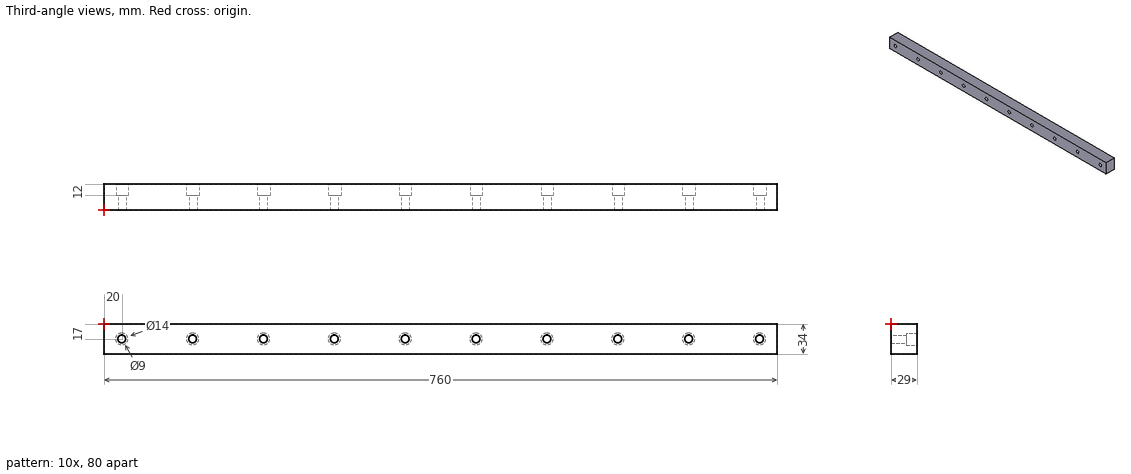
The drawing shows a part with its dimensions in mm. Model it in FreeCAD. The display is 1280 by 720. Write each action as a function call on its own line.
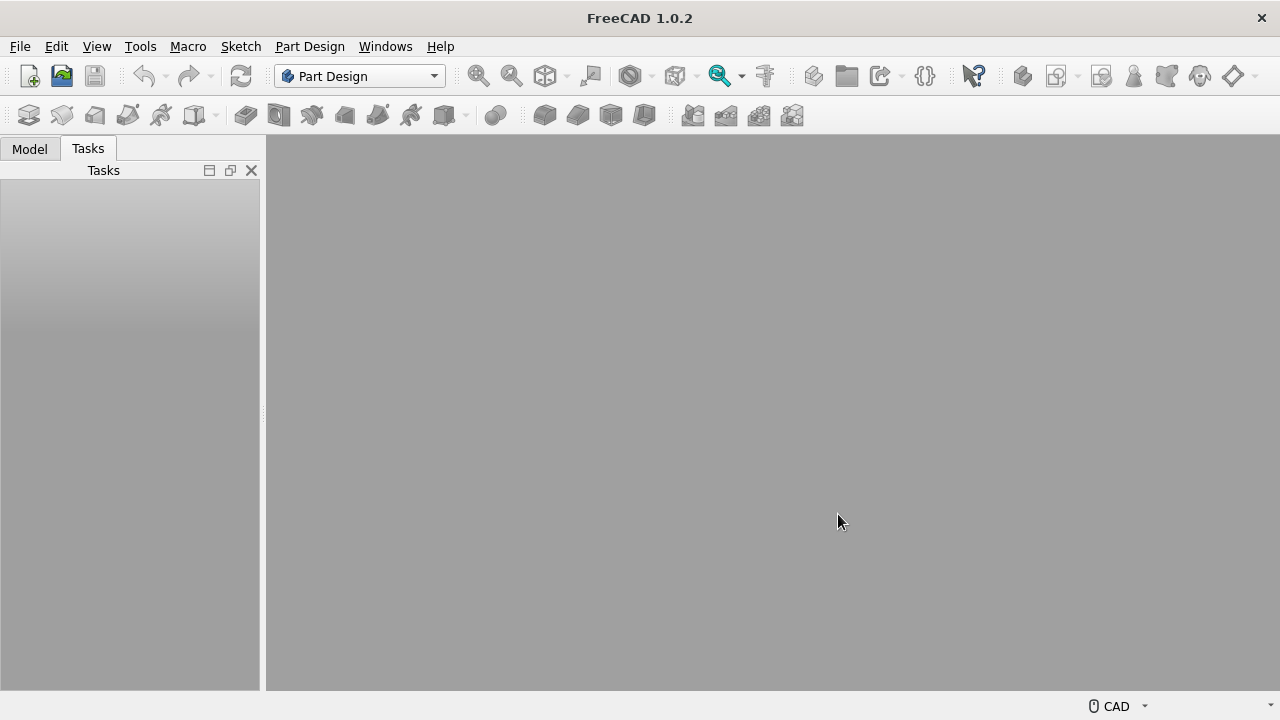
key(ctrl+n)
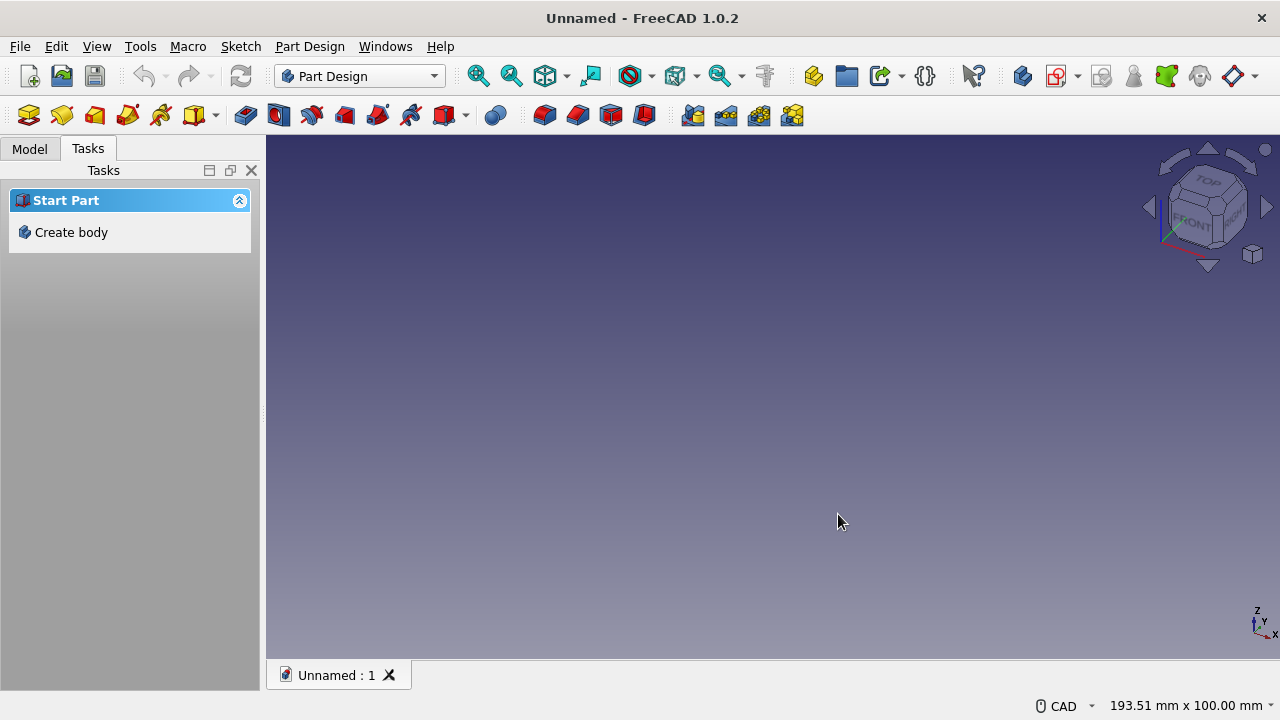
click(1056, 76)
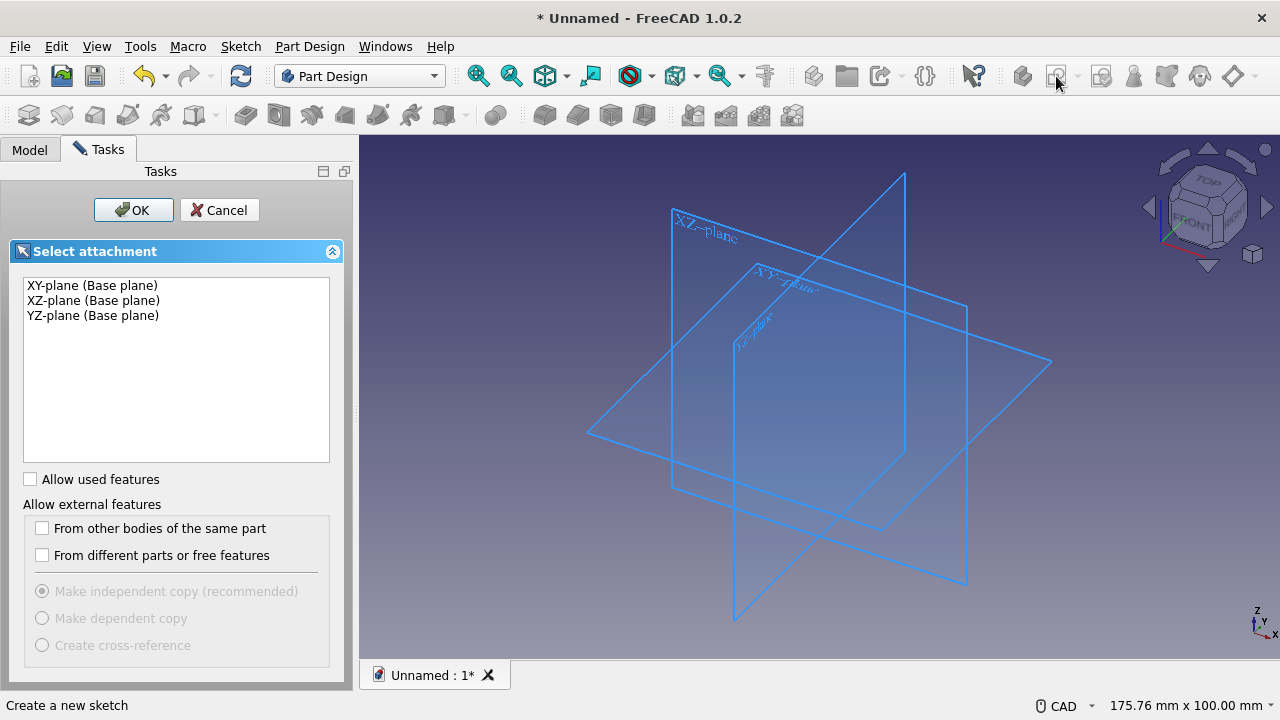
click(84, 300)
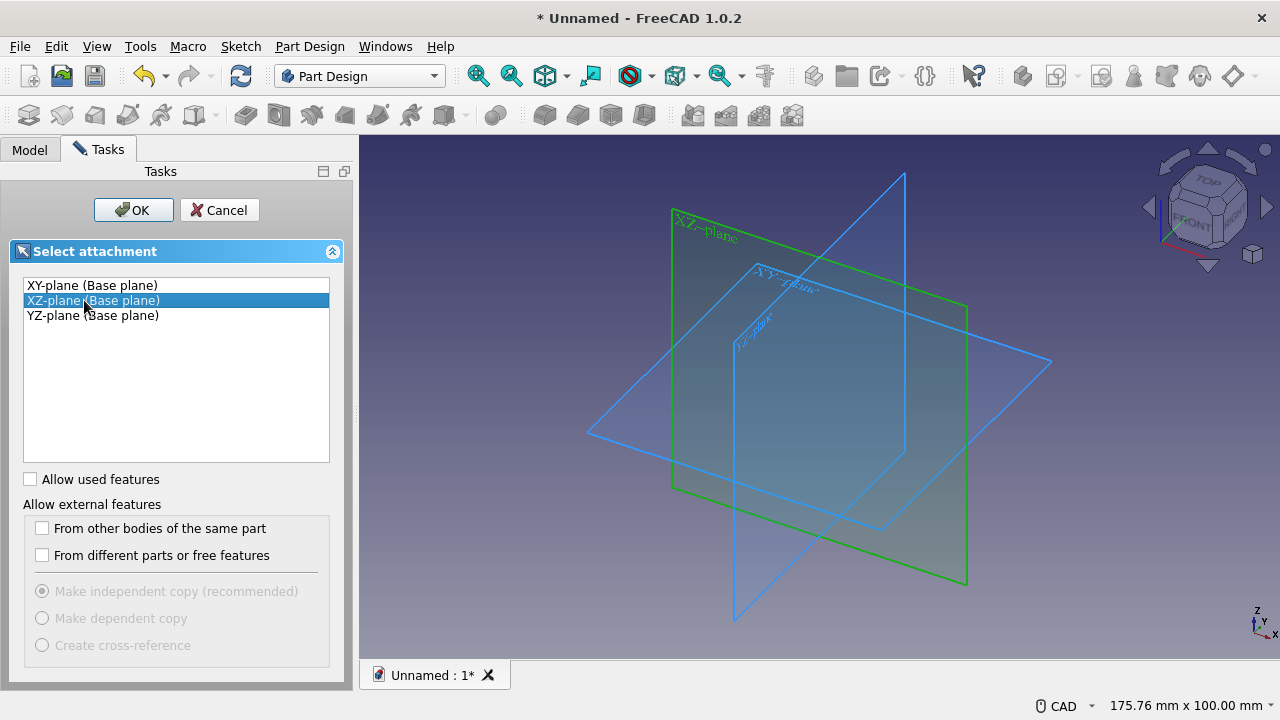
click(134, 210)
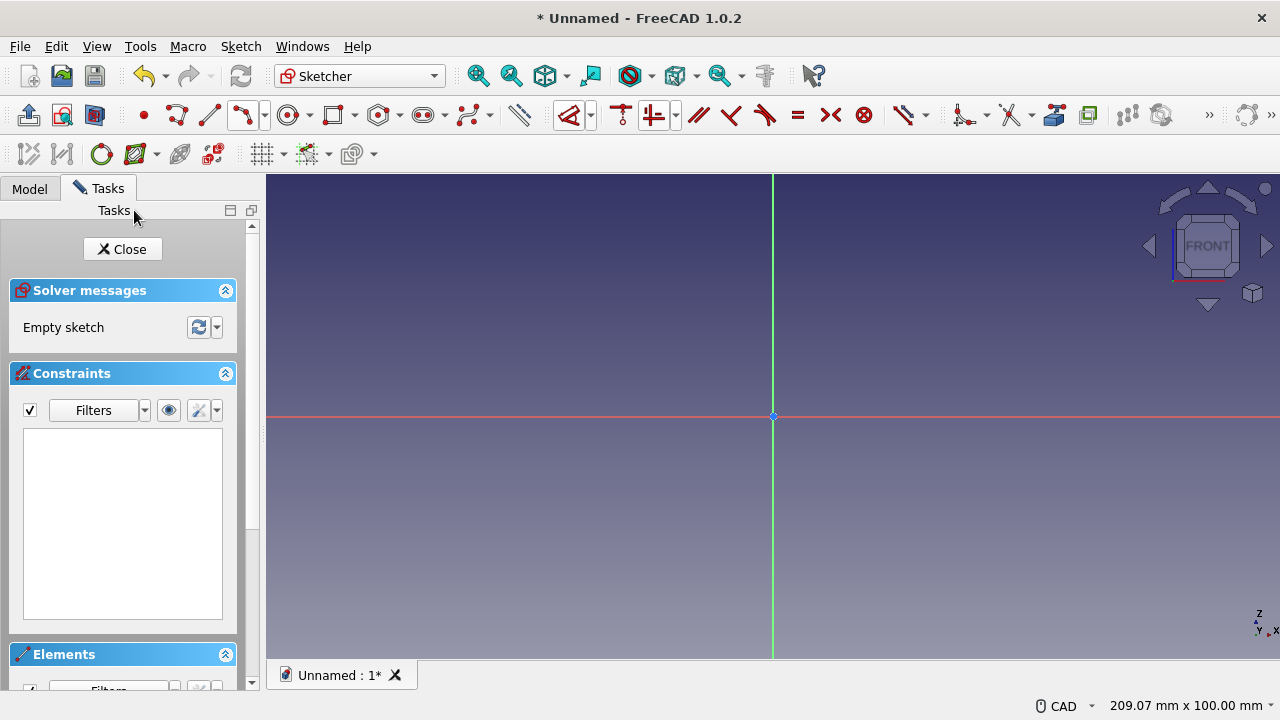
scroll(326, 400, down, 9)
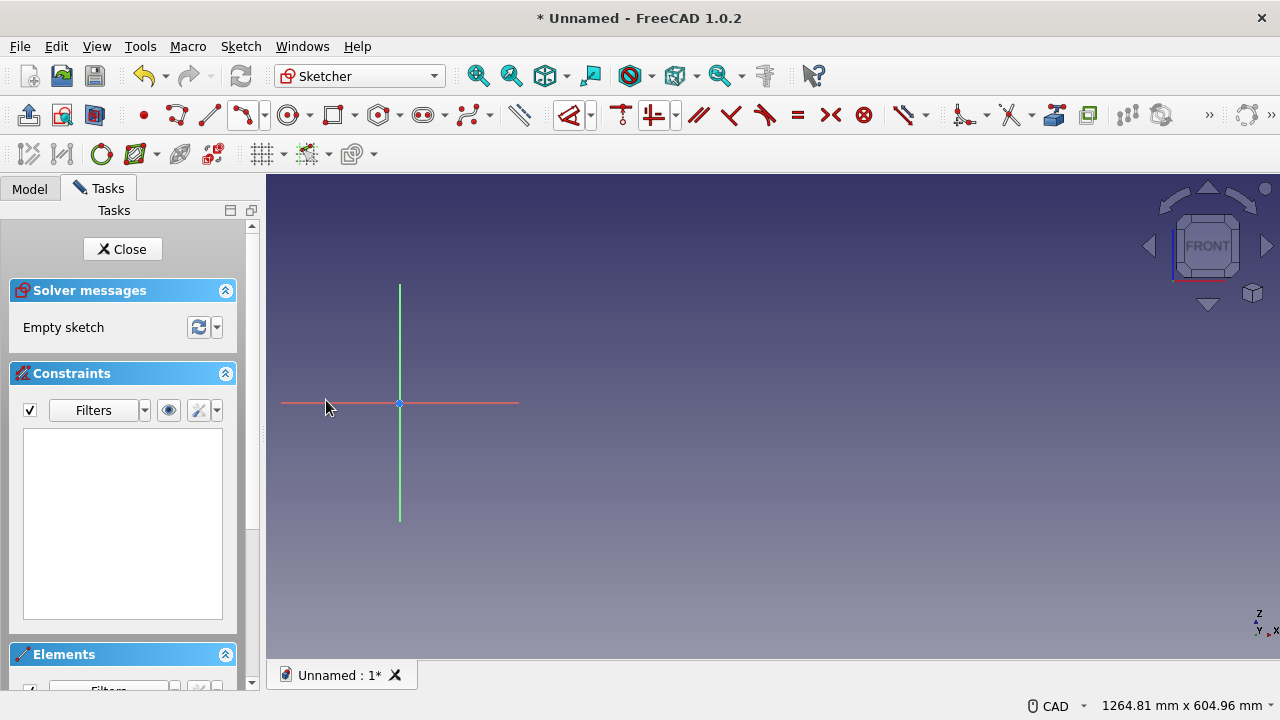
click(332, 116)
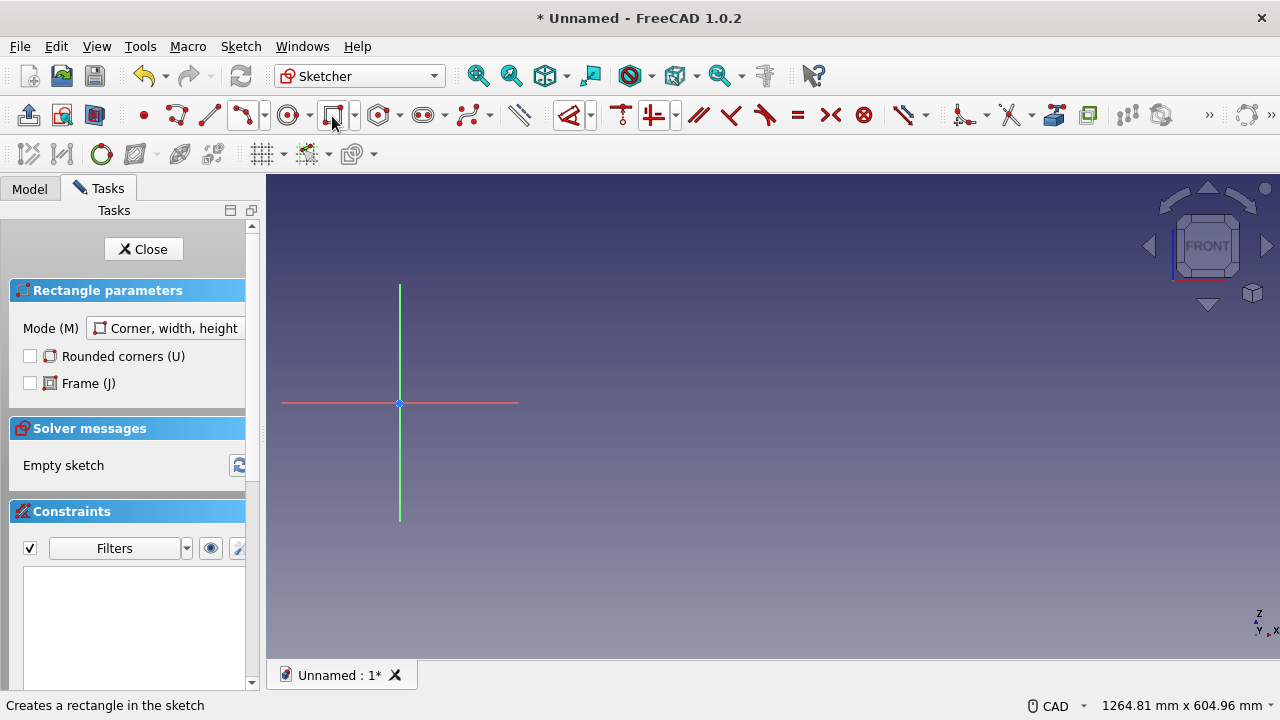
click(400, 403)
move(1009, 430)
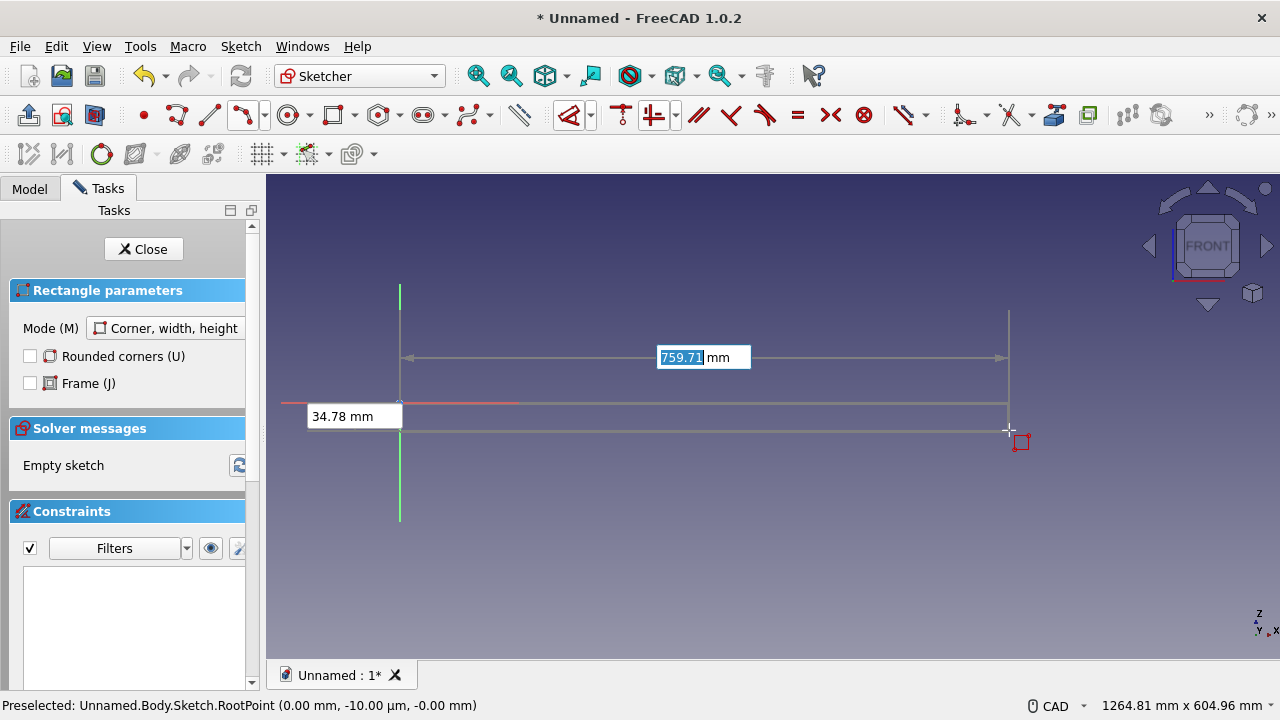
text(760)
key(Tab)
text(34)
key(Return)
key(Escape)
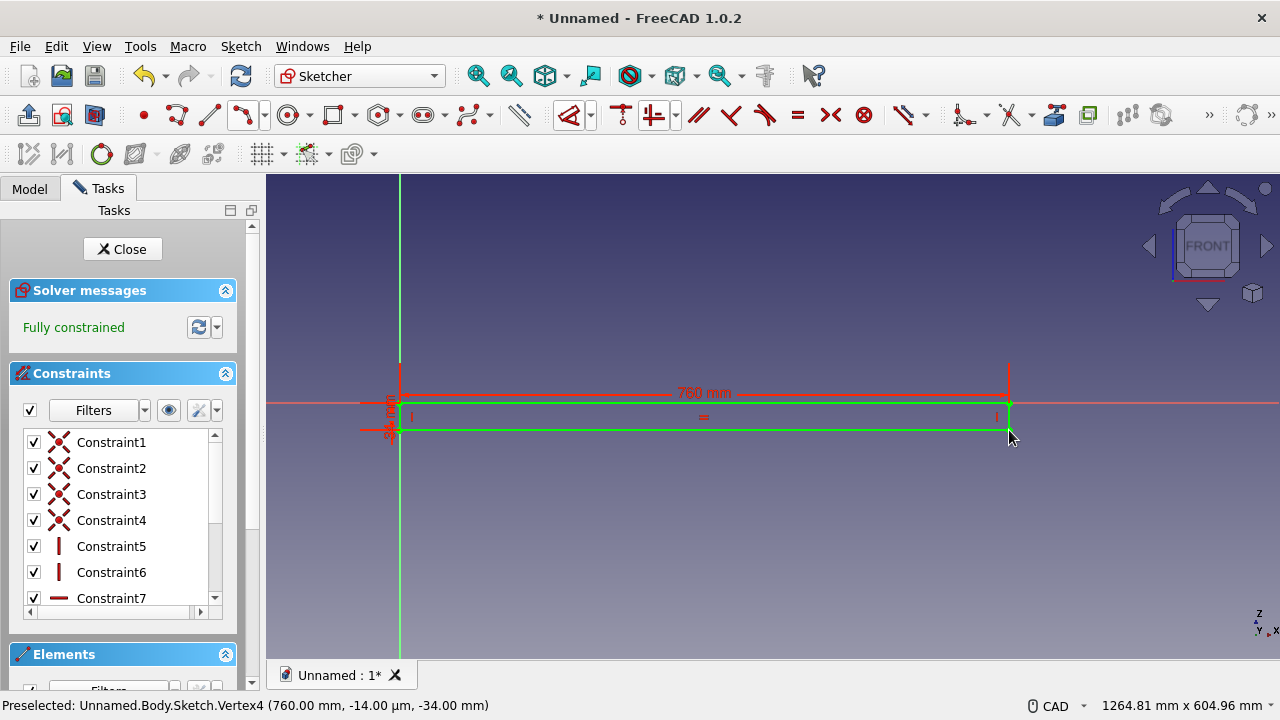
click(123, 249)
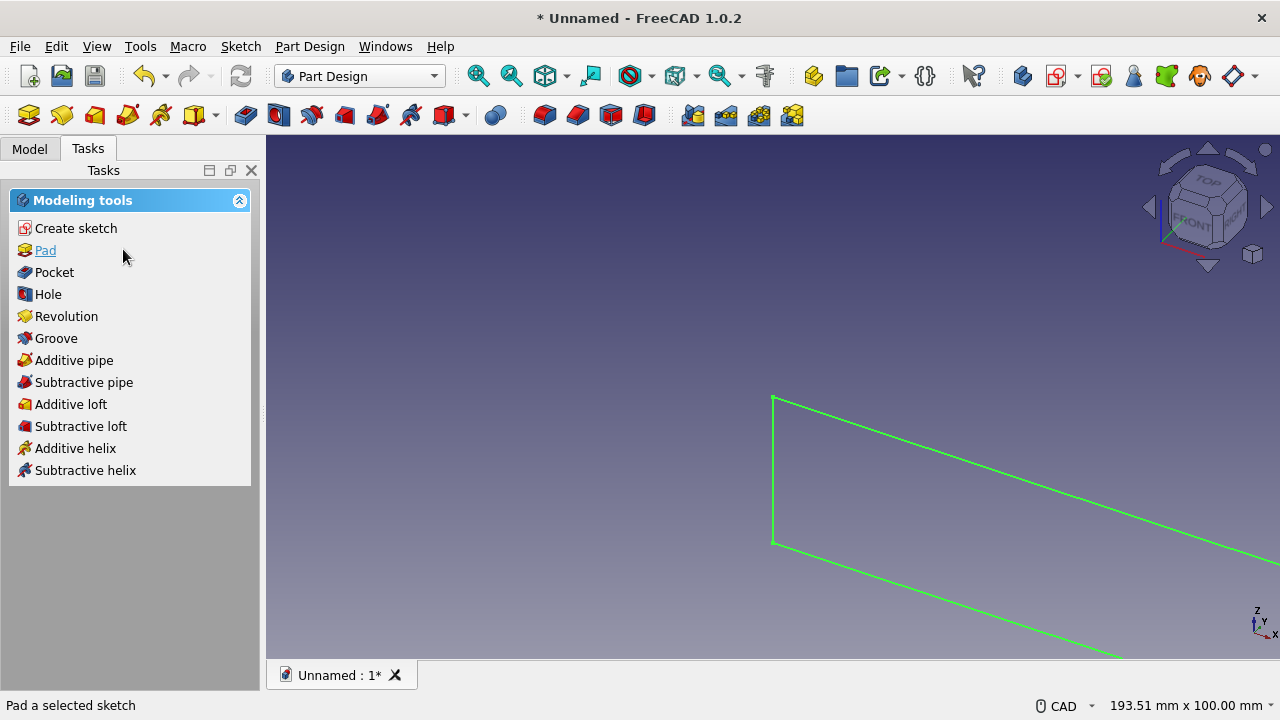
click(29, 116)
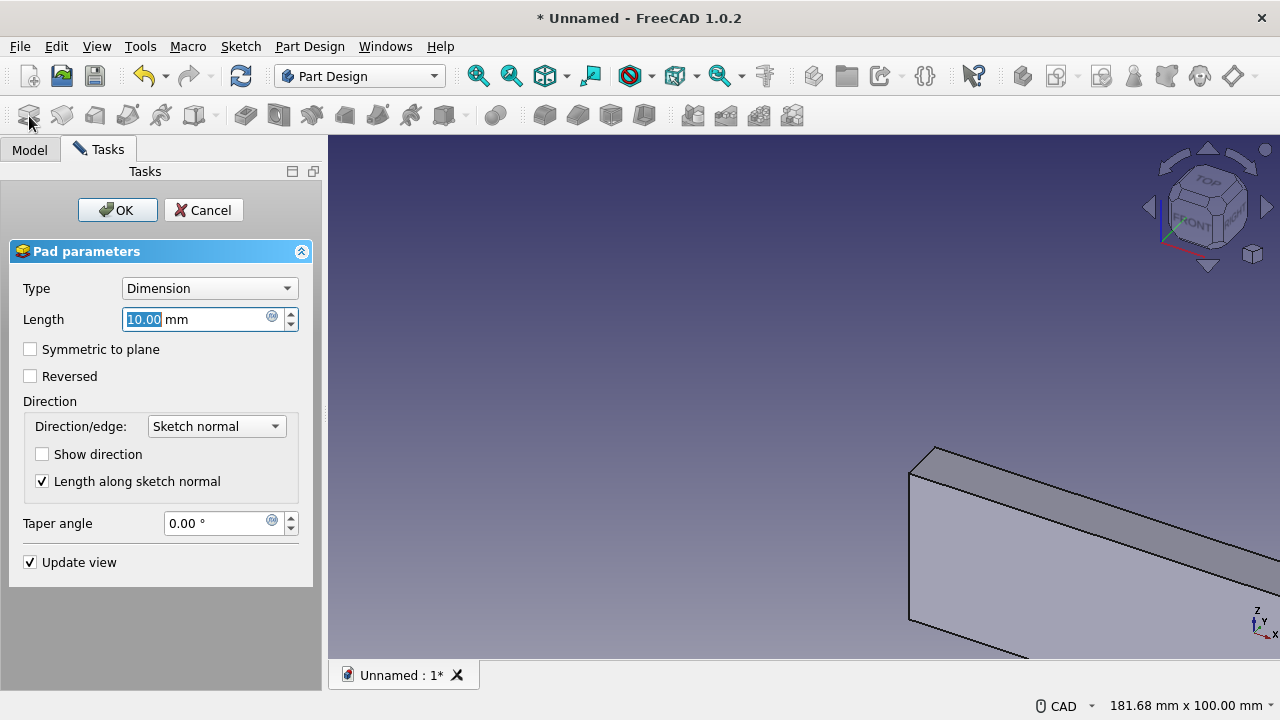
text(29)
key(Tab)